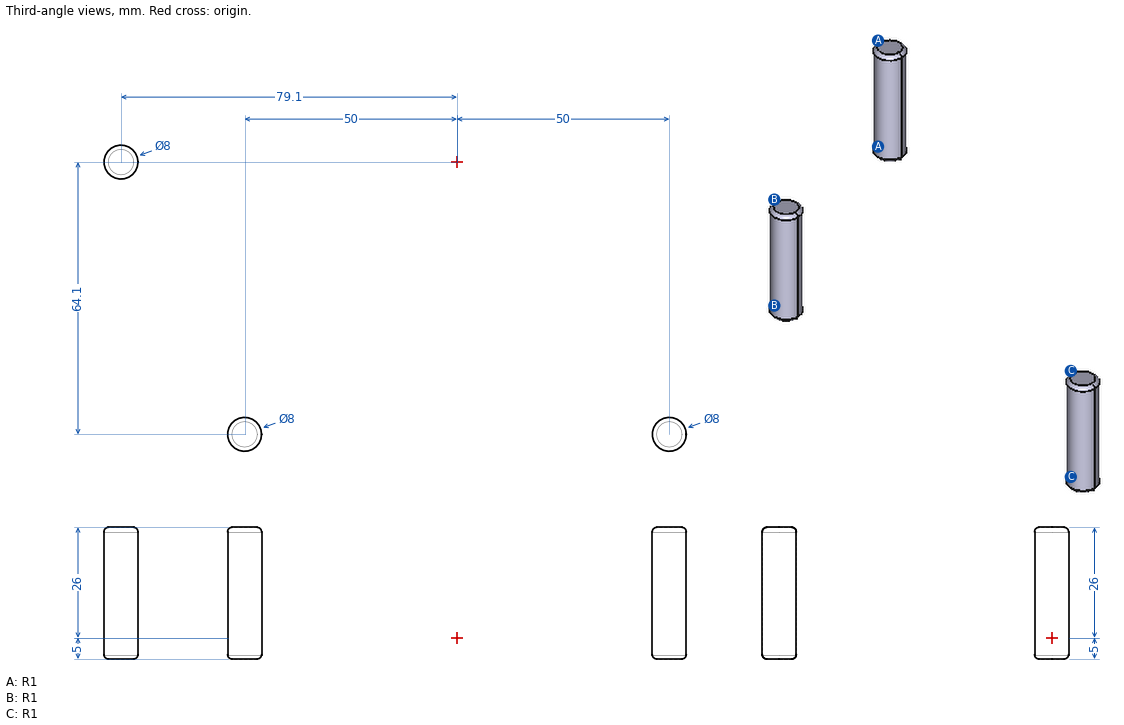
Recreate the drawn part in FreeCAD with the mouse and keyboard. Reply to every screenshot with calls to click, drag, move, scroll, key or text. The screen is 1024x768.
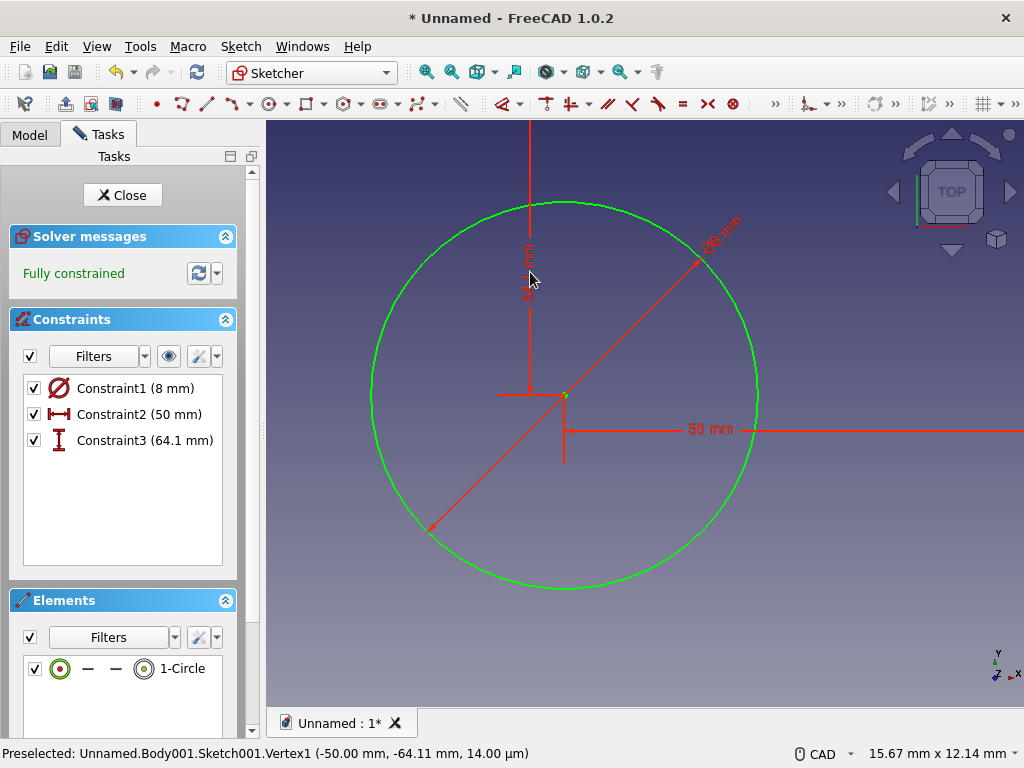
click(123, 195)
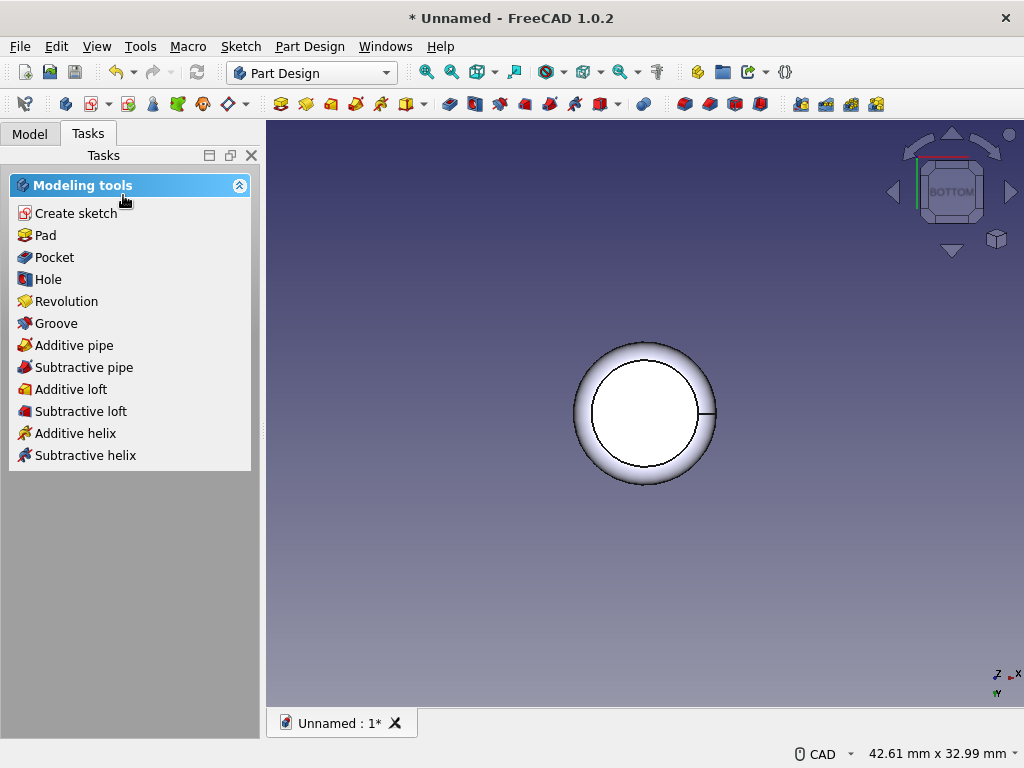
click(281, 104)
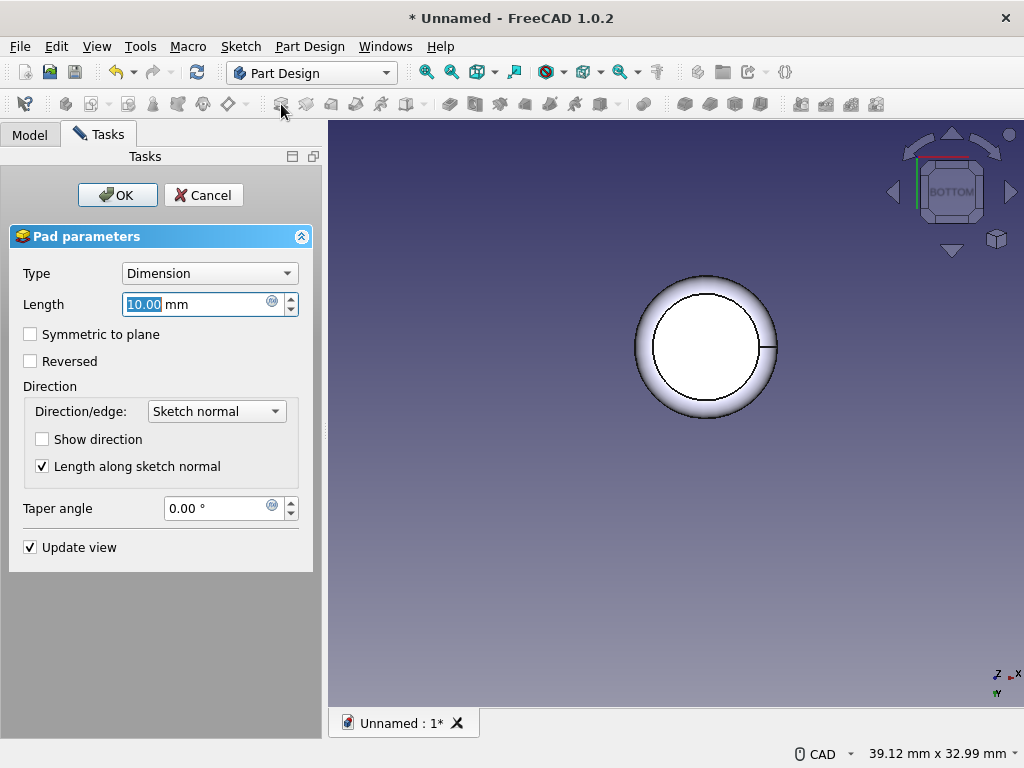
click(210, 274)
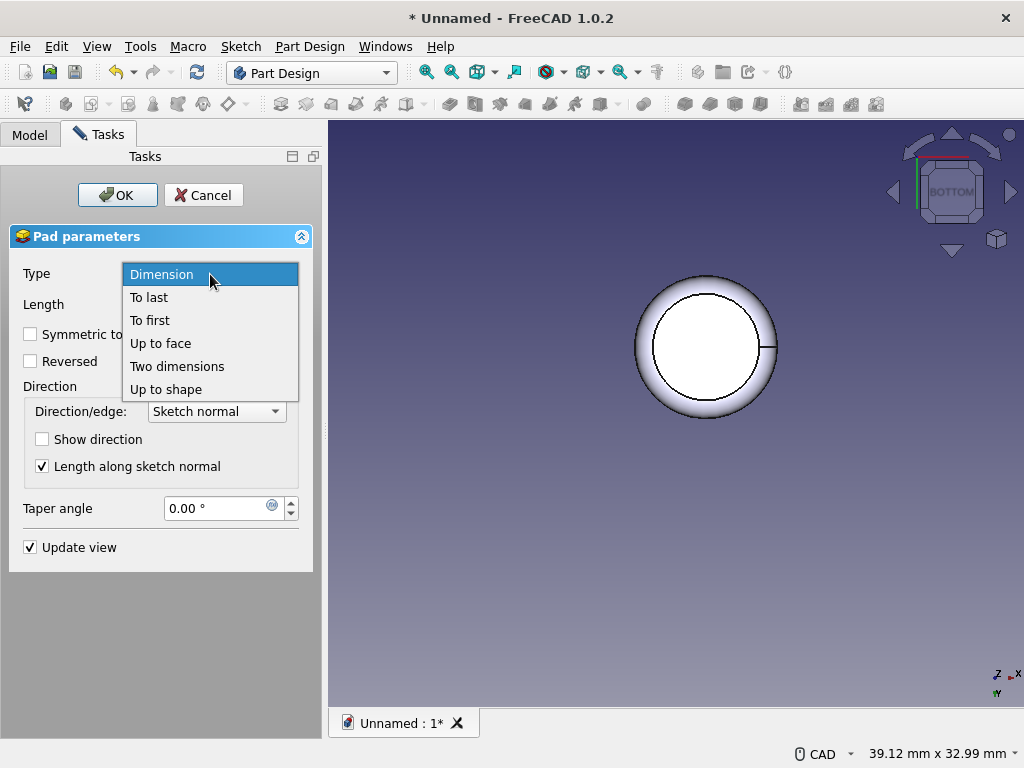
click(208, 366)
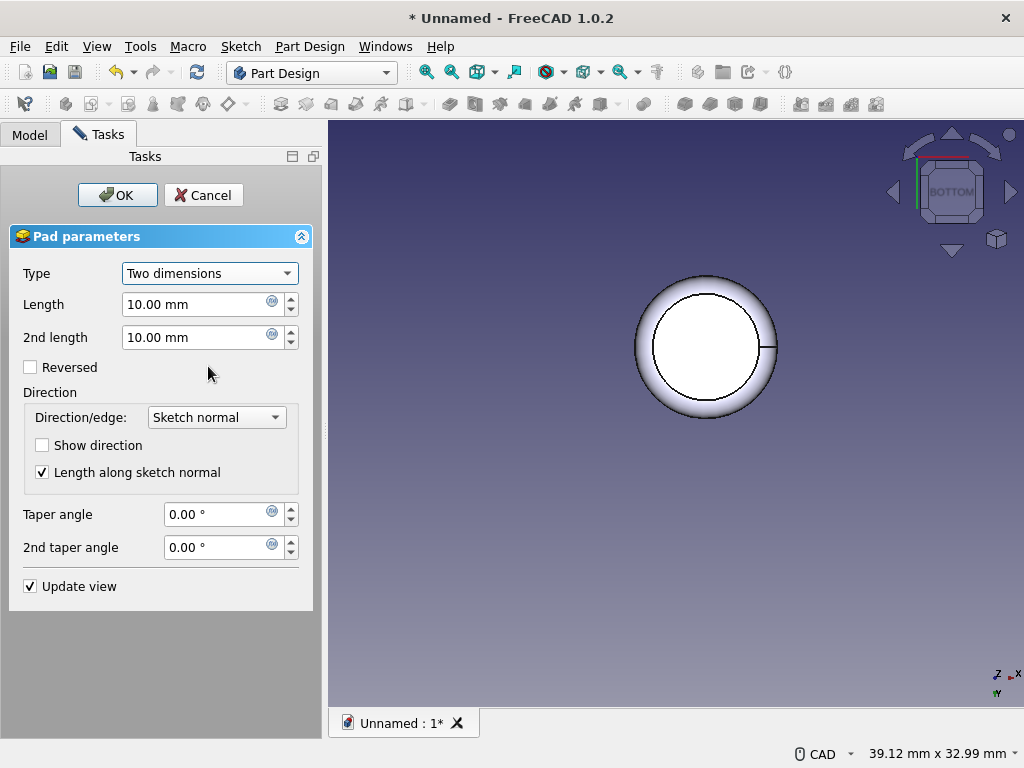
triple_click(204, 304)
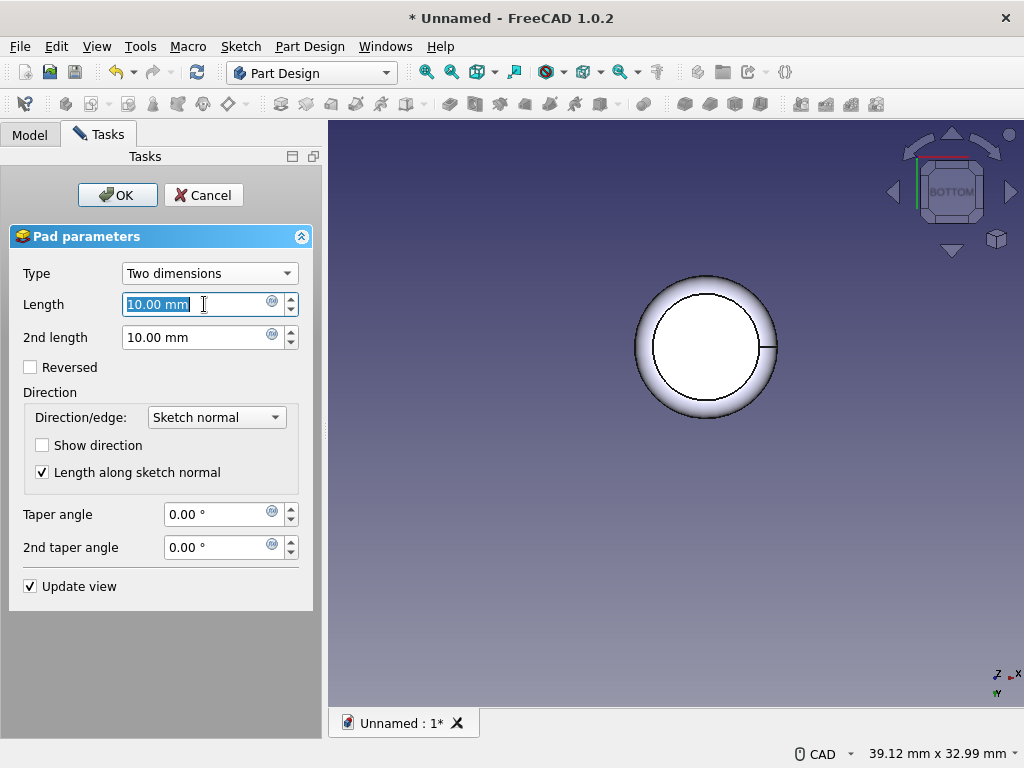
text(26)
key(Tab)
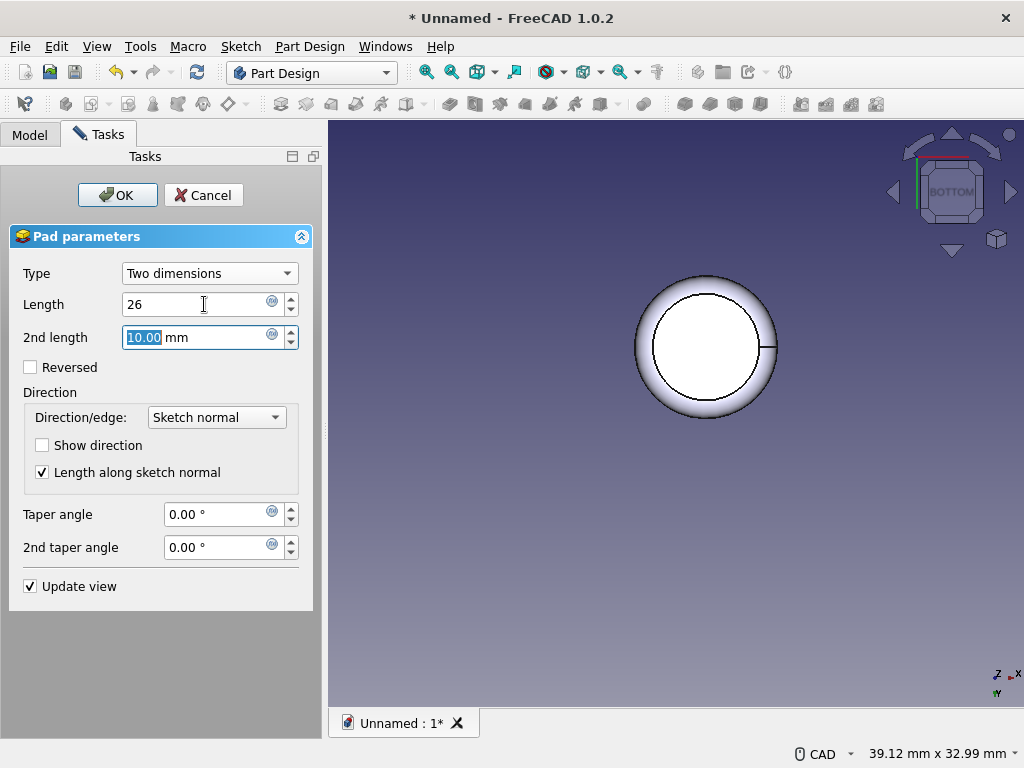
text(5)
key(Tab)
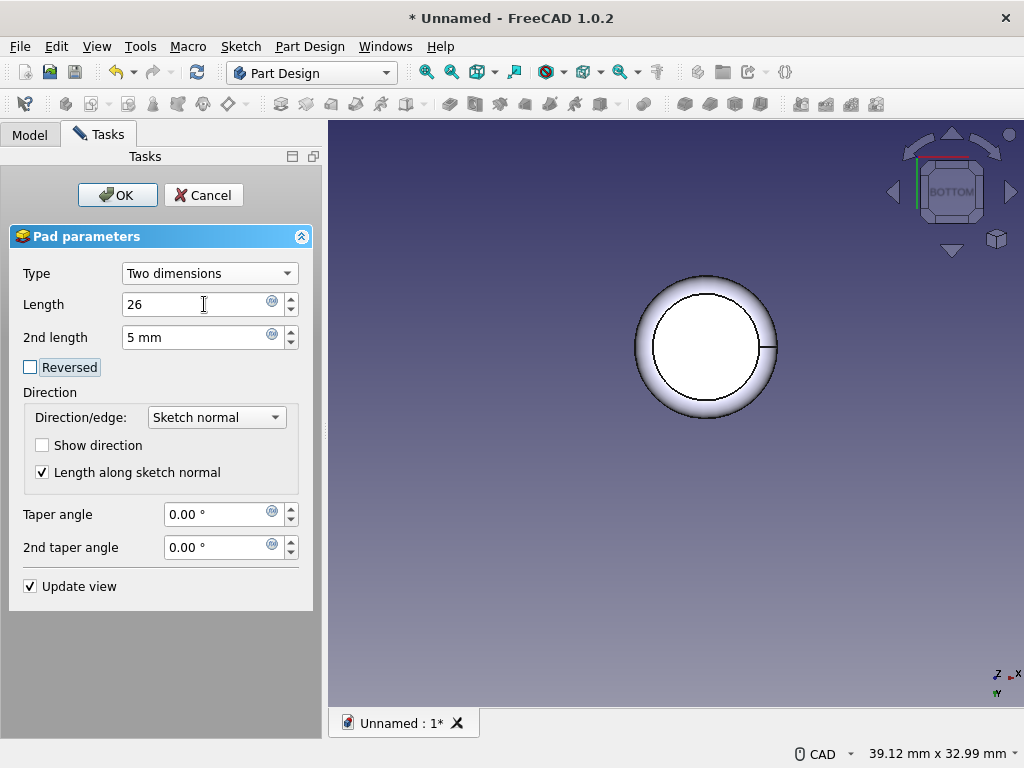
click(118, 195)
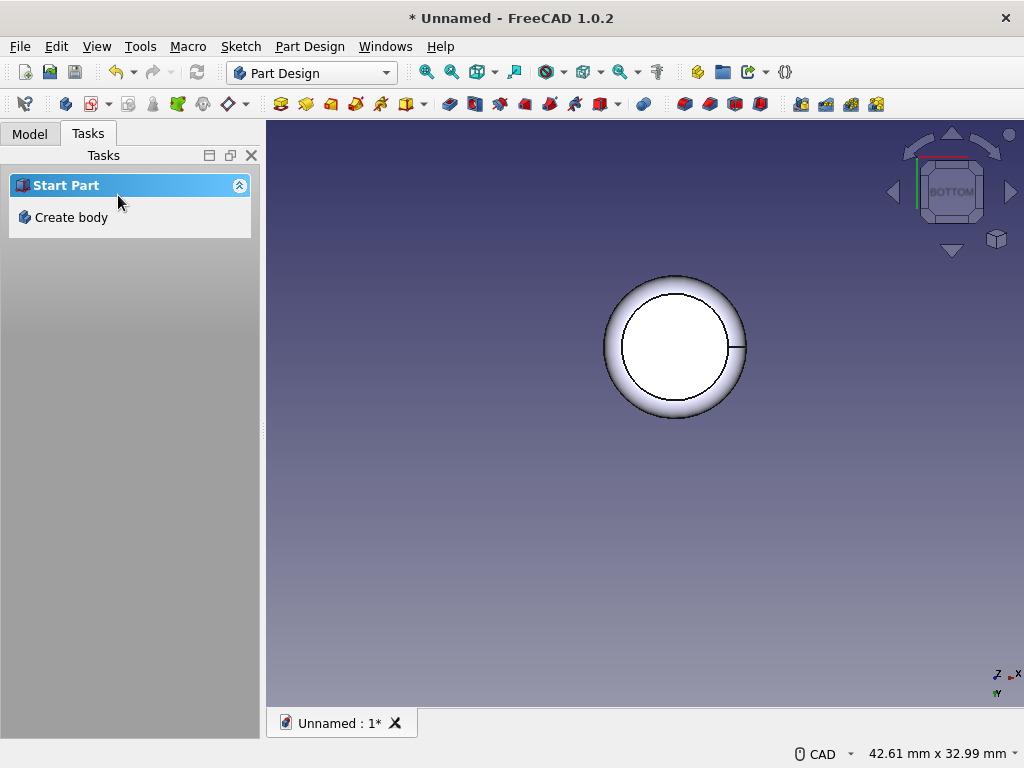
click(427, 72)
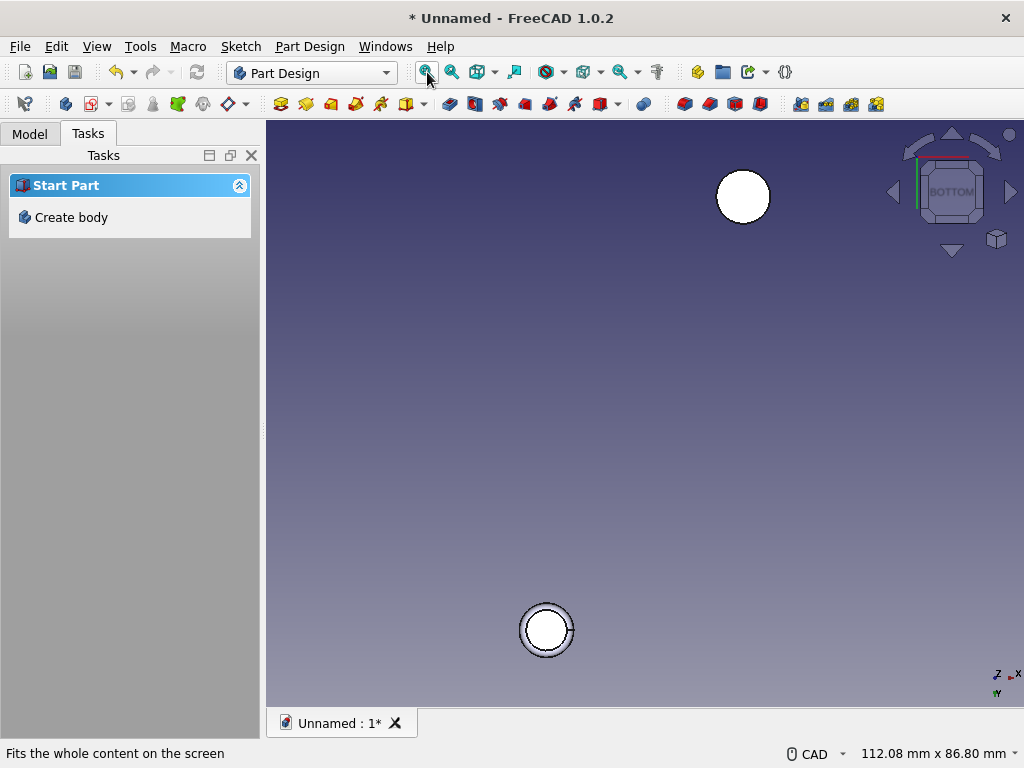
click(716, 196)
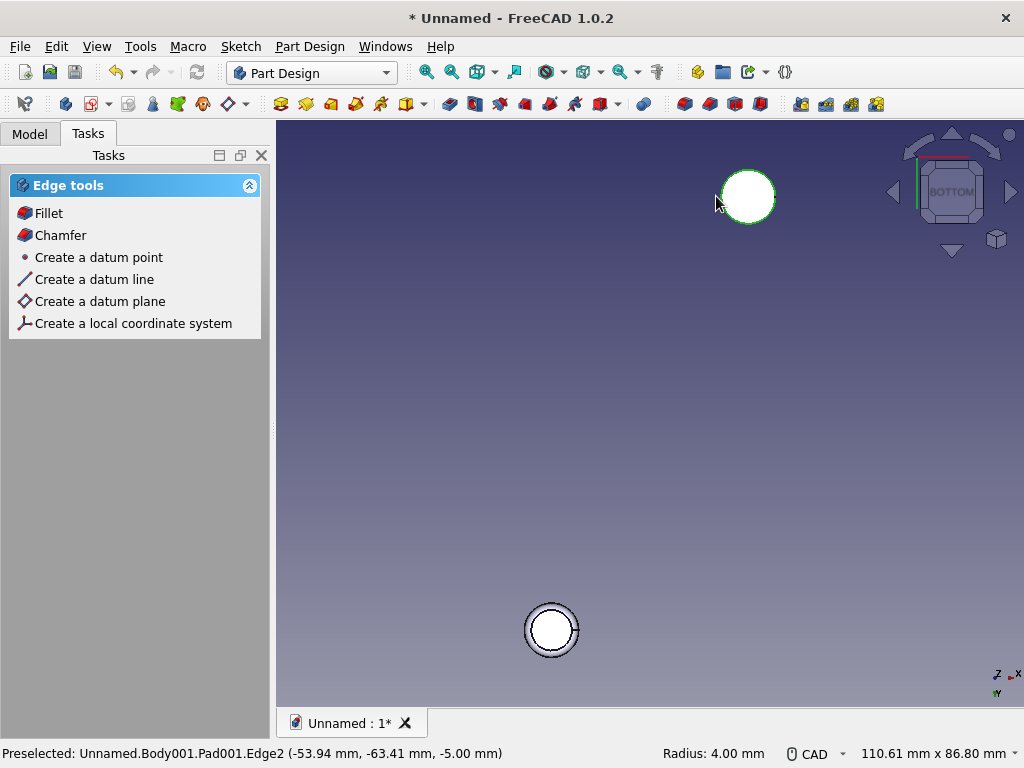
key(0)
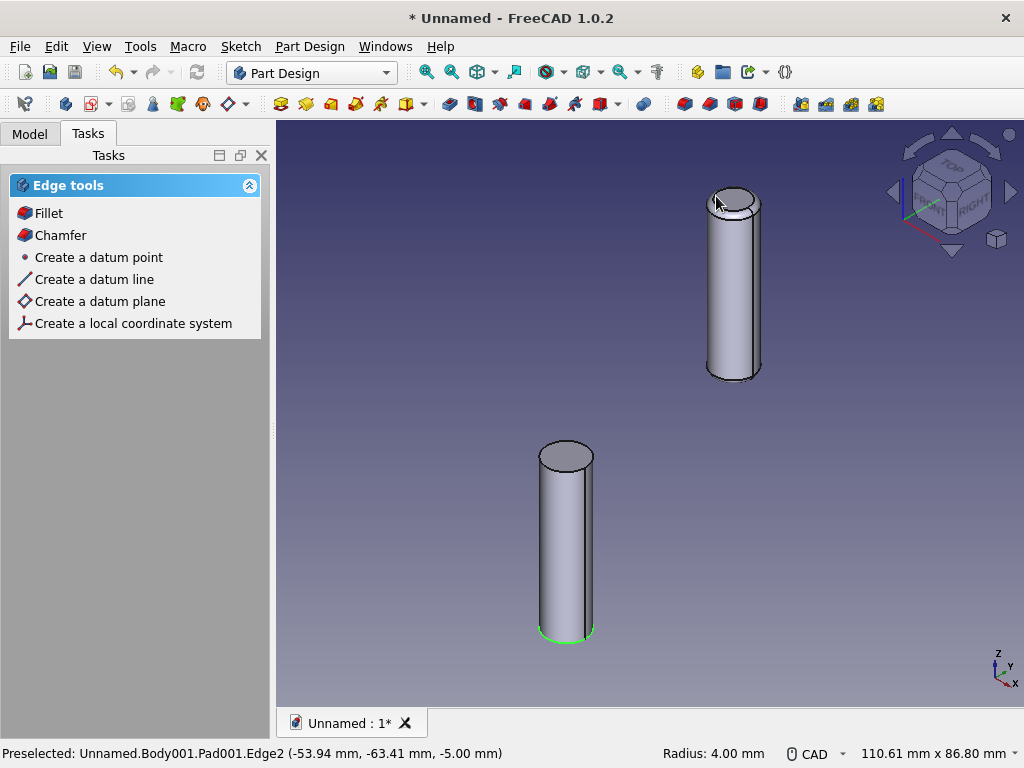
click(427, 72)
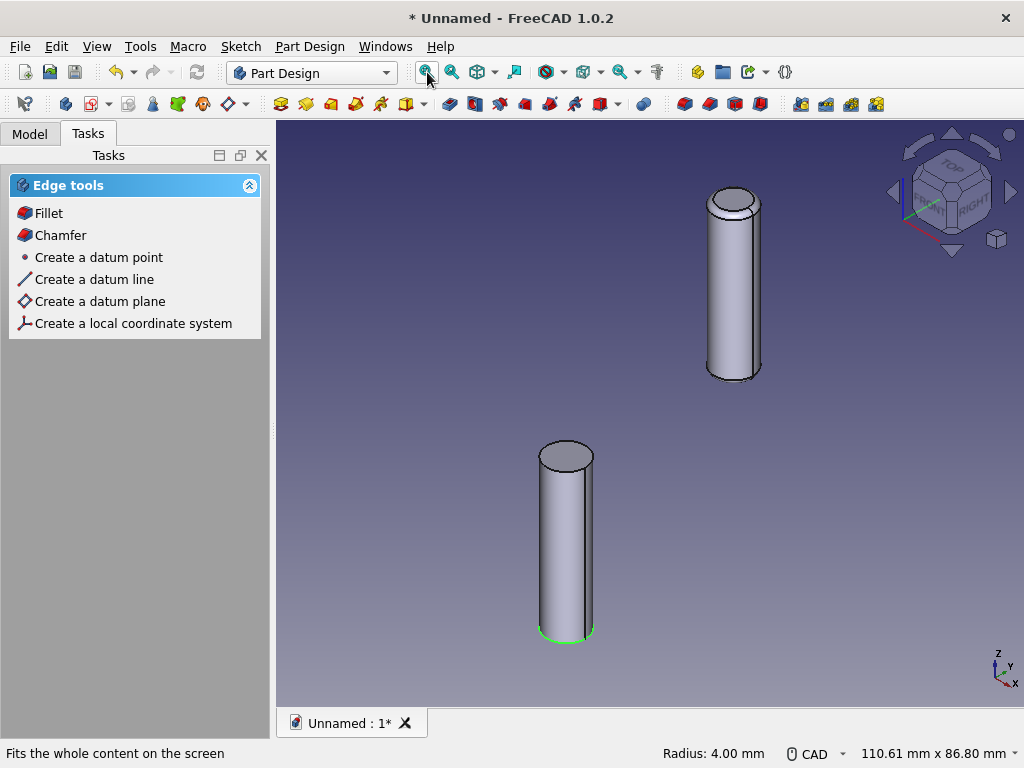
click(540, 453, ctrl)